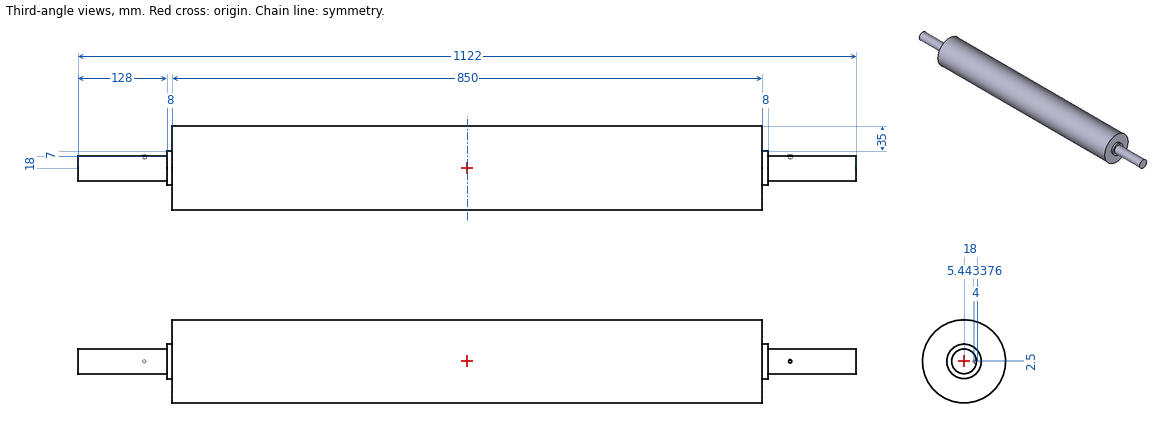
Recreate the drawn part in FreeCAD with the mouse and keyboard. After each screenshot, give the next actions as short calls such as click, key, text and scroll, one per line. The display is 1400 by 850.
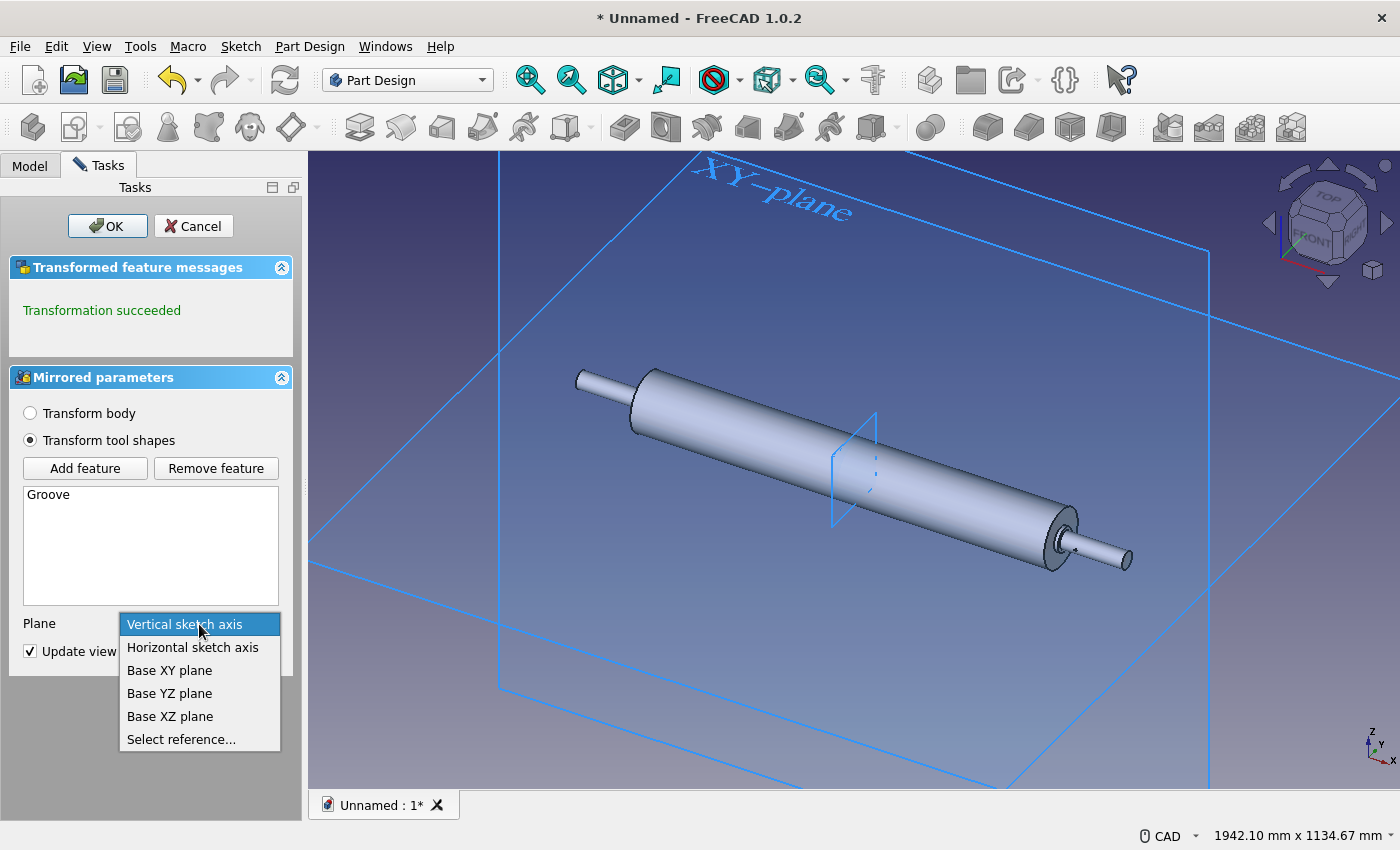
click(198, 694)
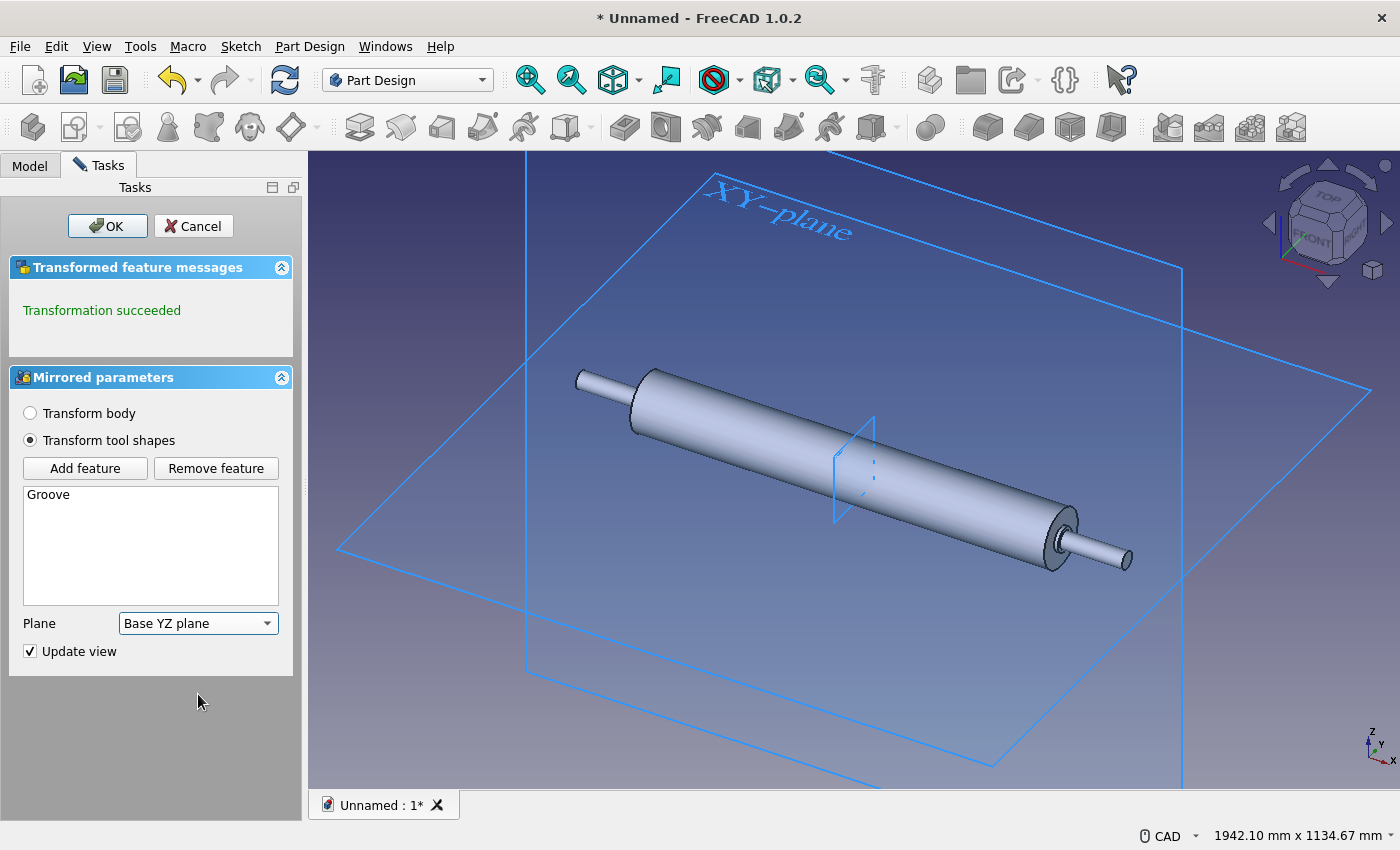
click(108, 226)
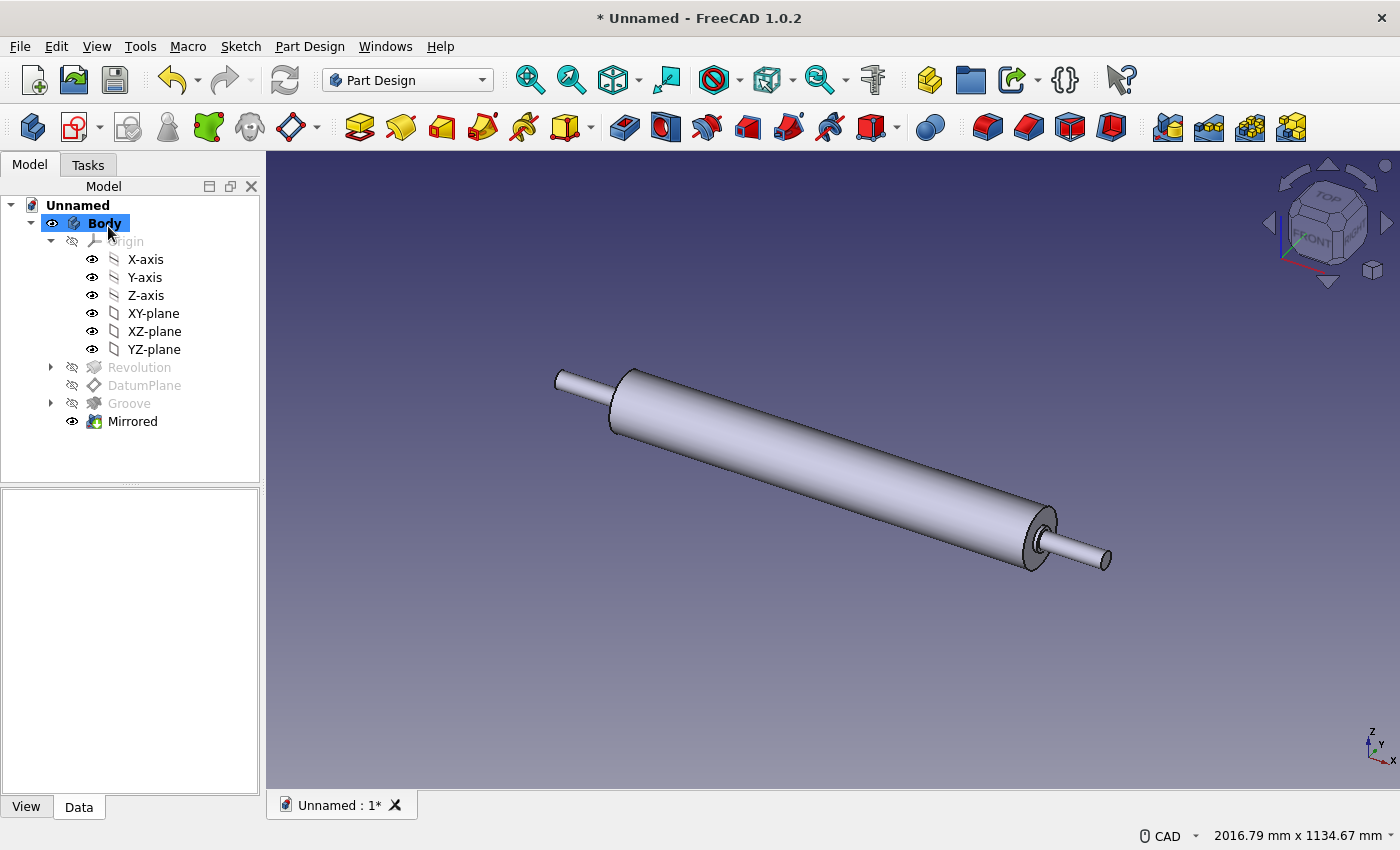
key(0)